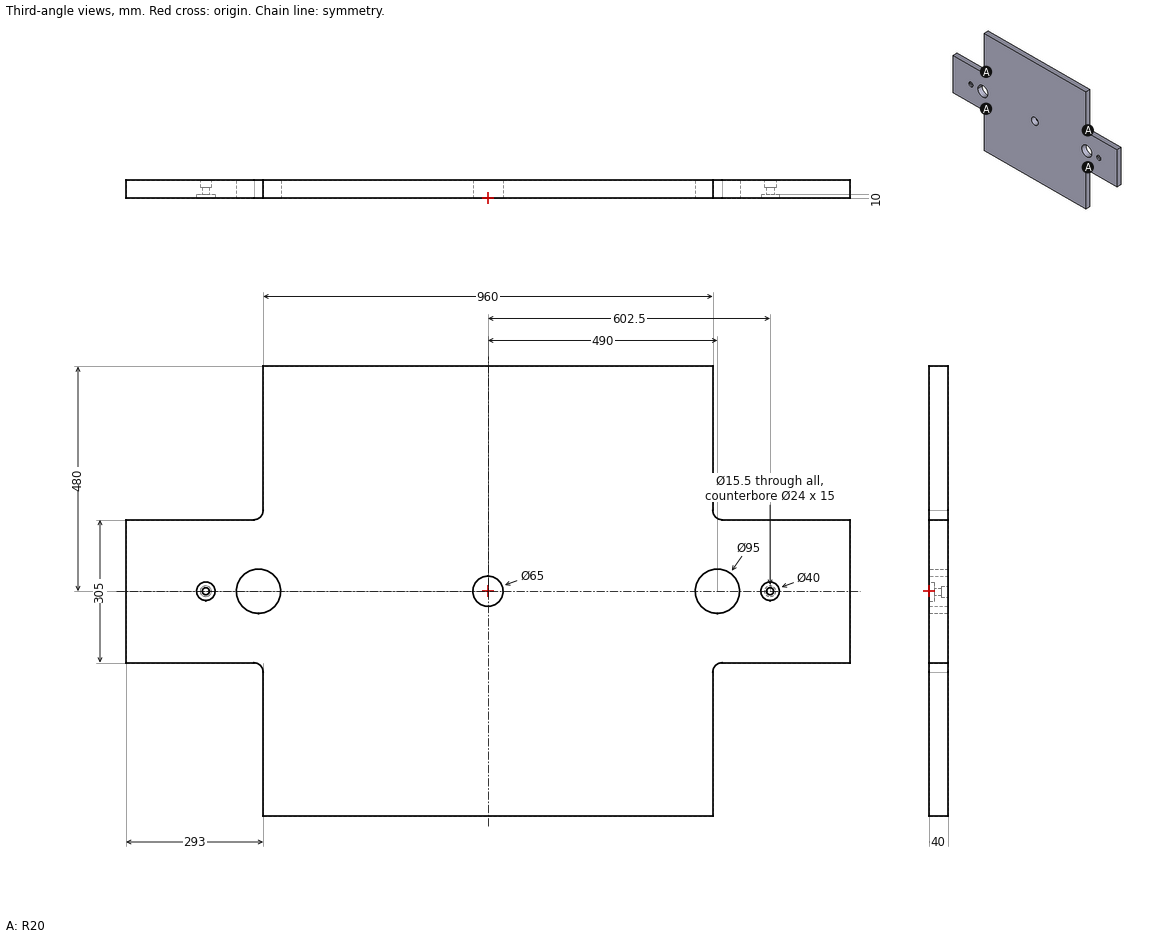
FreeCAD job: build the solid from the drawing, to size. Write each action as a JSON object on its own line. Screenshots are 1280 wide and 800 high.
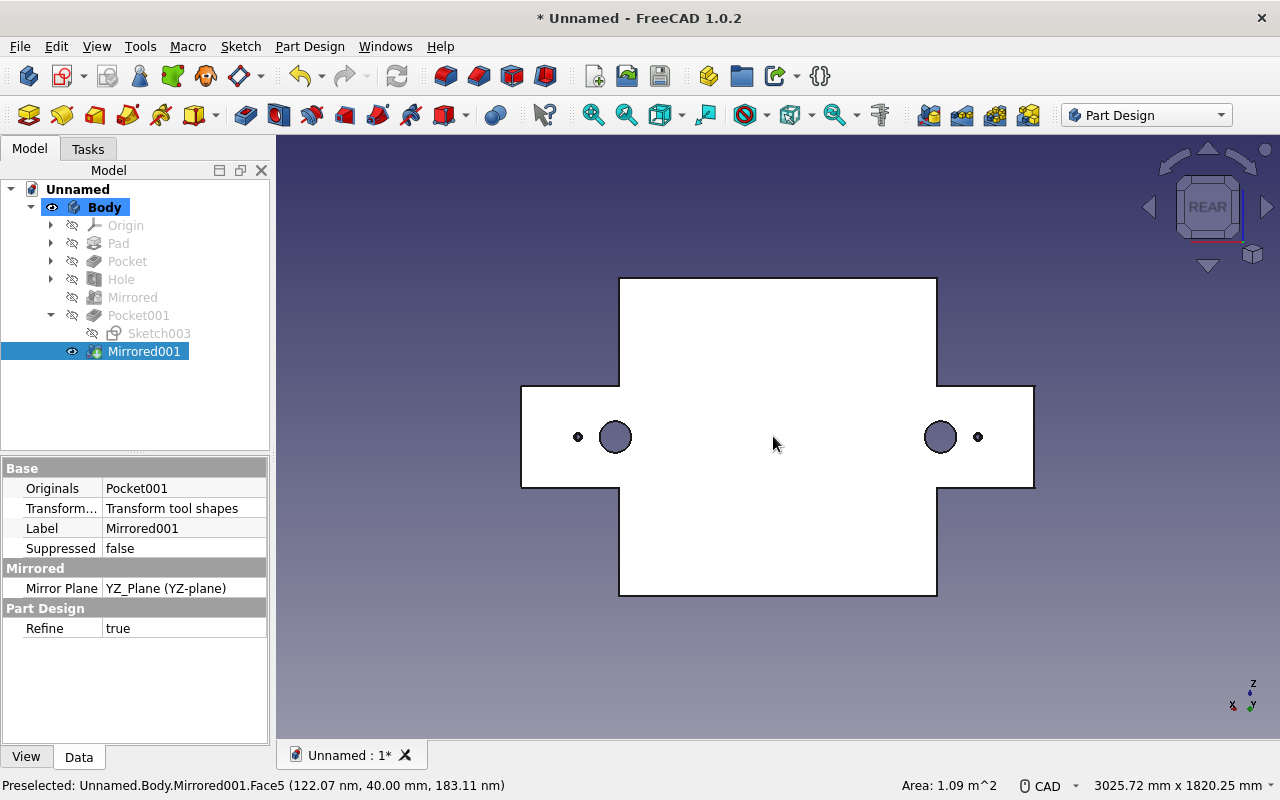
{"action": "left_click", "coordinate": [62, 76]}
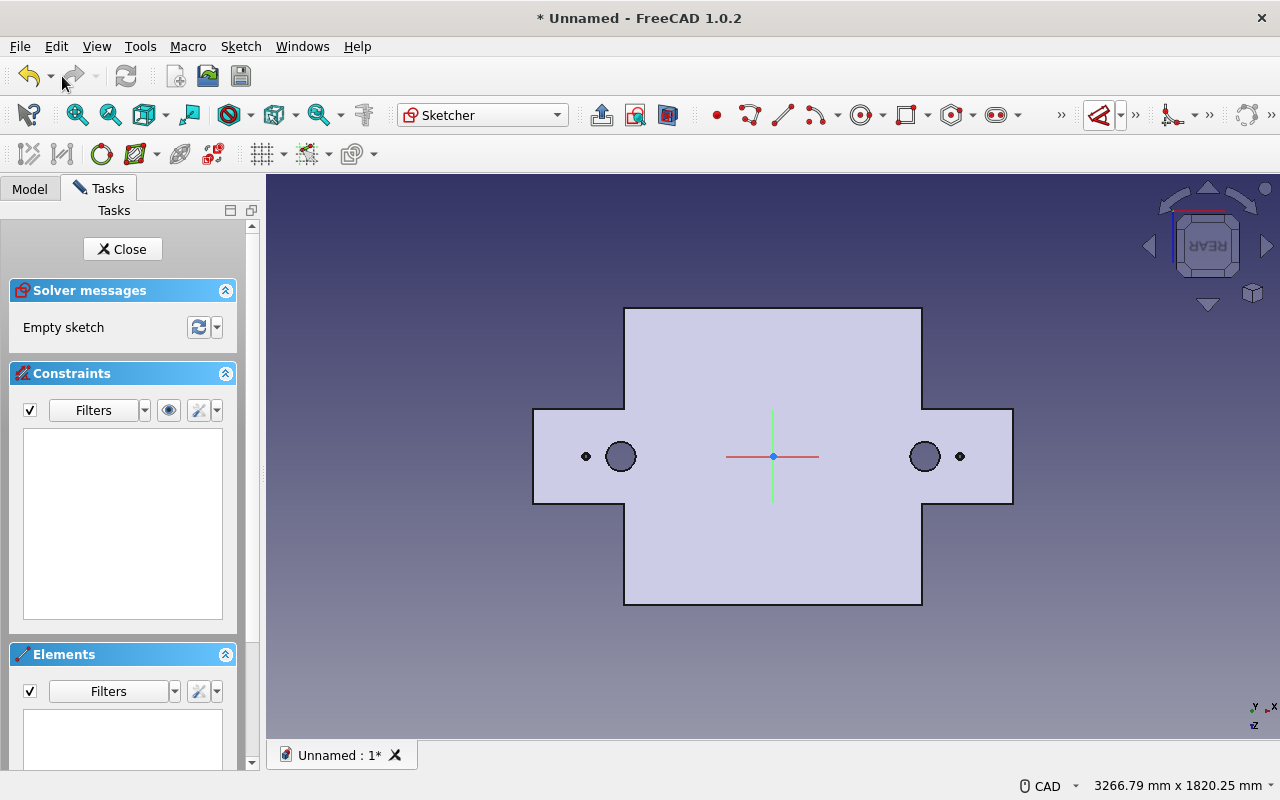
{"action": "scroll", "coordinate": [777, 456], "scroll_direction": "up", "scroll_amount": 14}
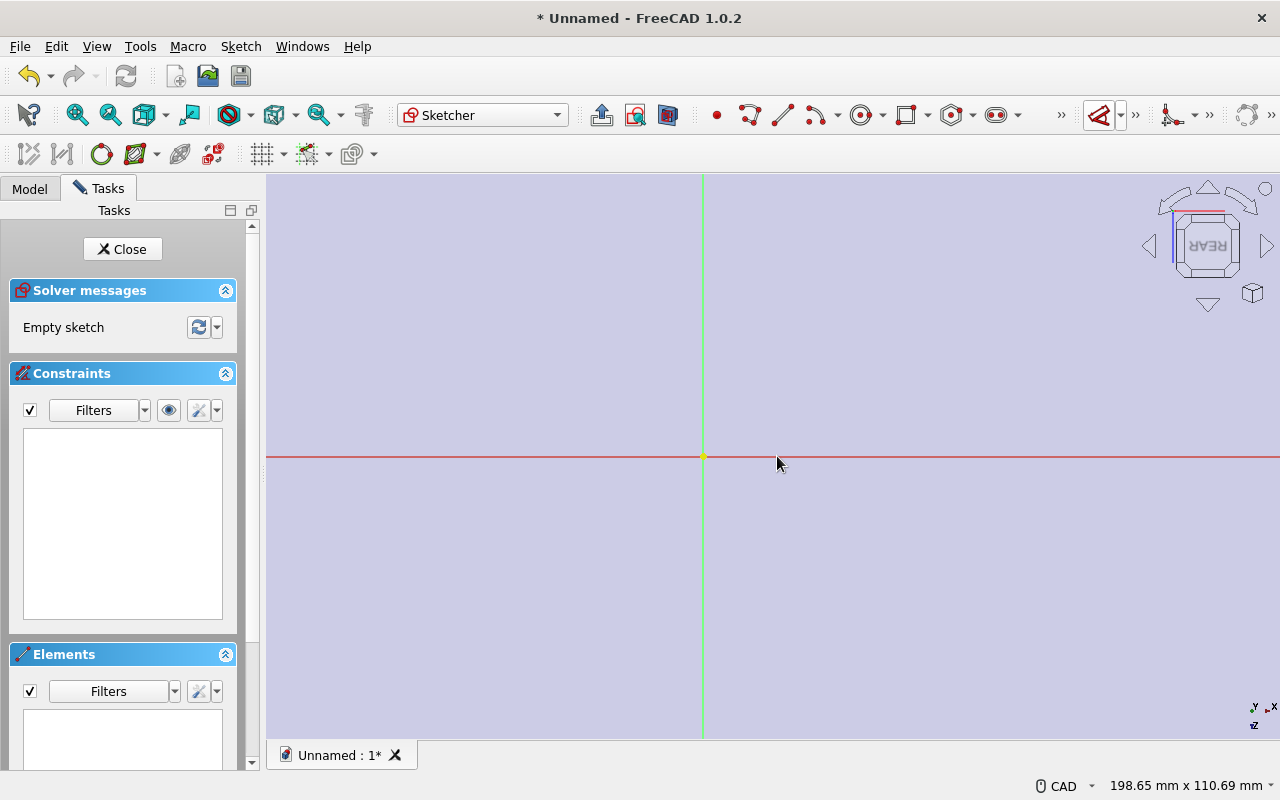
{"action": "left_click", "coordinate": [860, 116]}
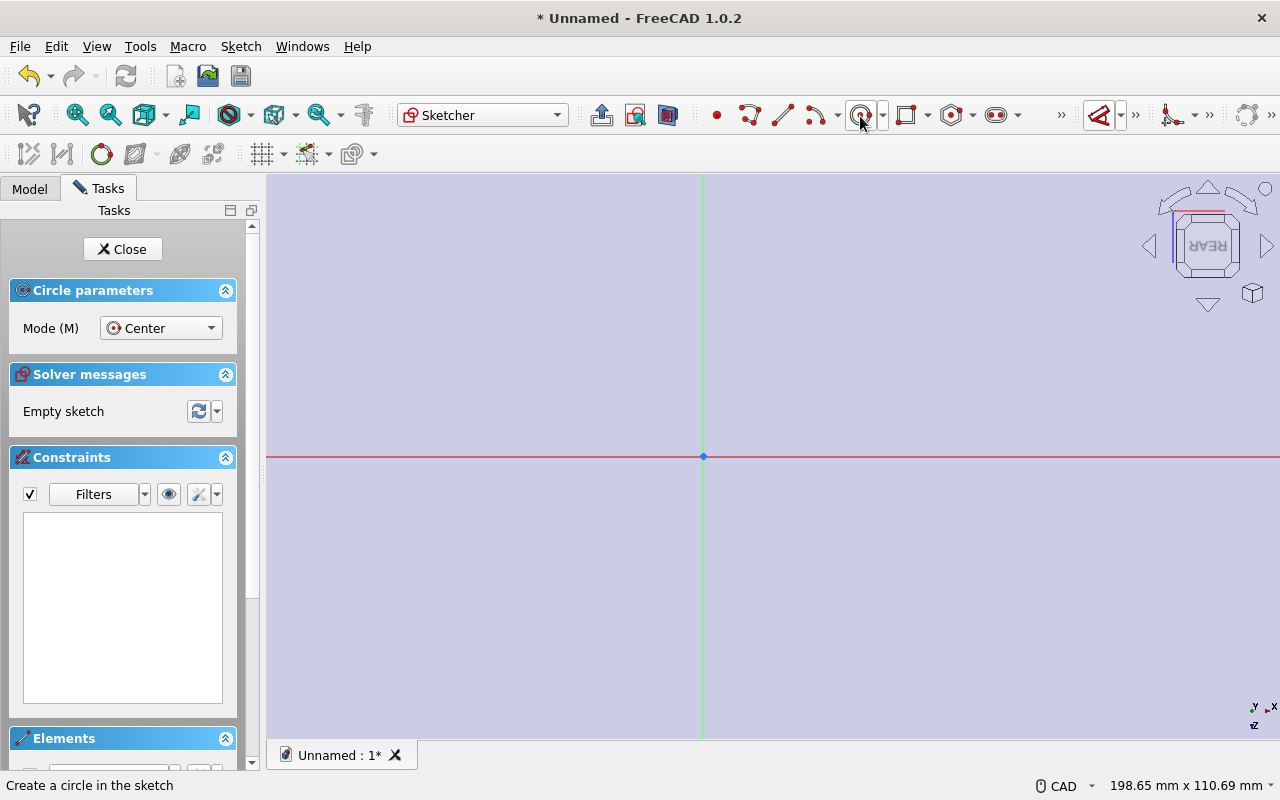
{"action": "left_click", "coordinate": [703, 456]}
{"action": "mouse_move", "coordinate": [821, 339]}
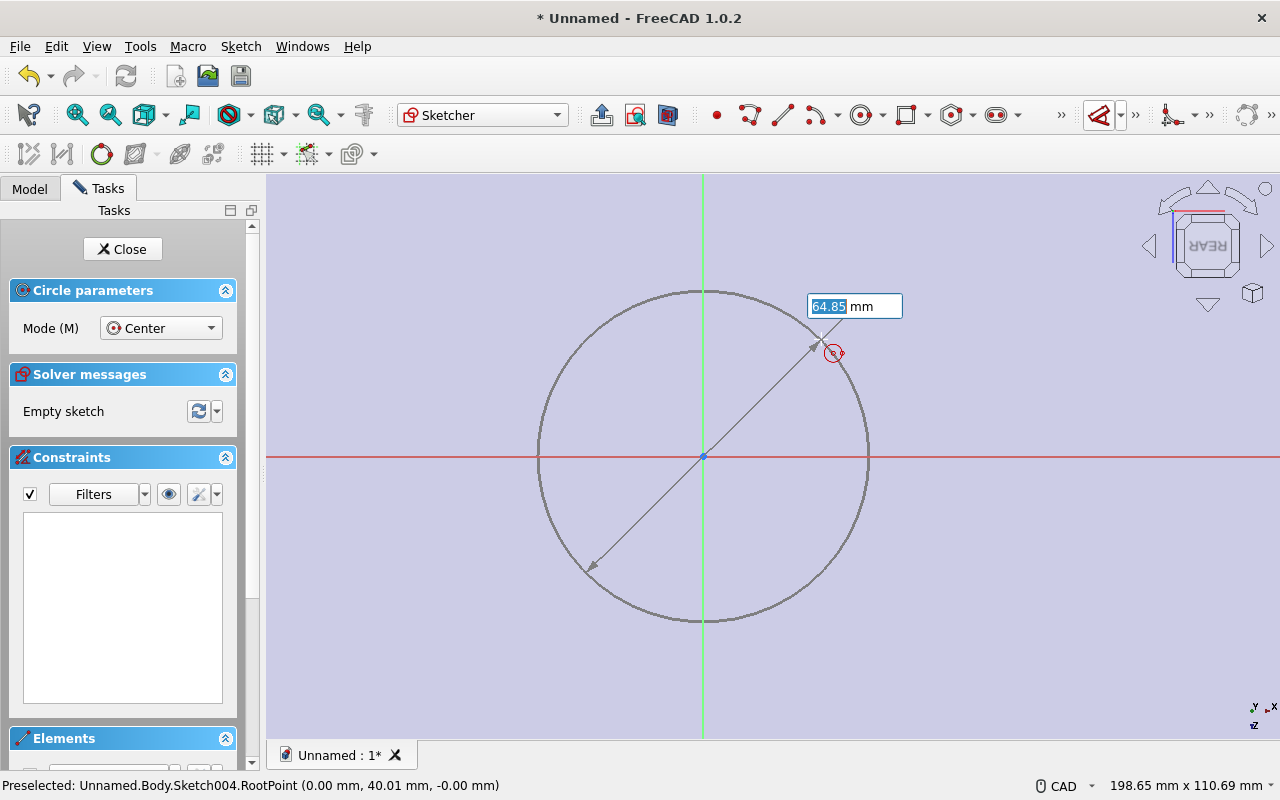
{"action": "type", "text": "65"}
{"action": "key", "text": "Return"}
{"action": "key", "text": "Escape"}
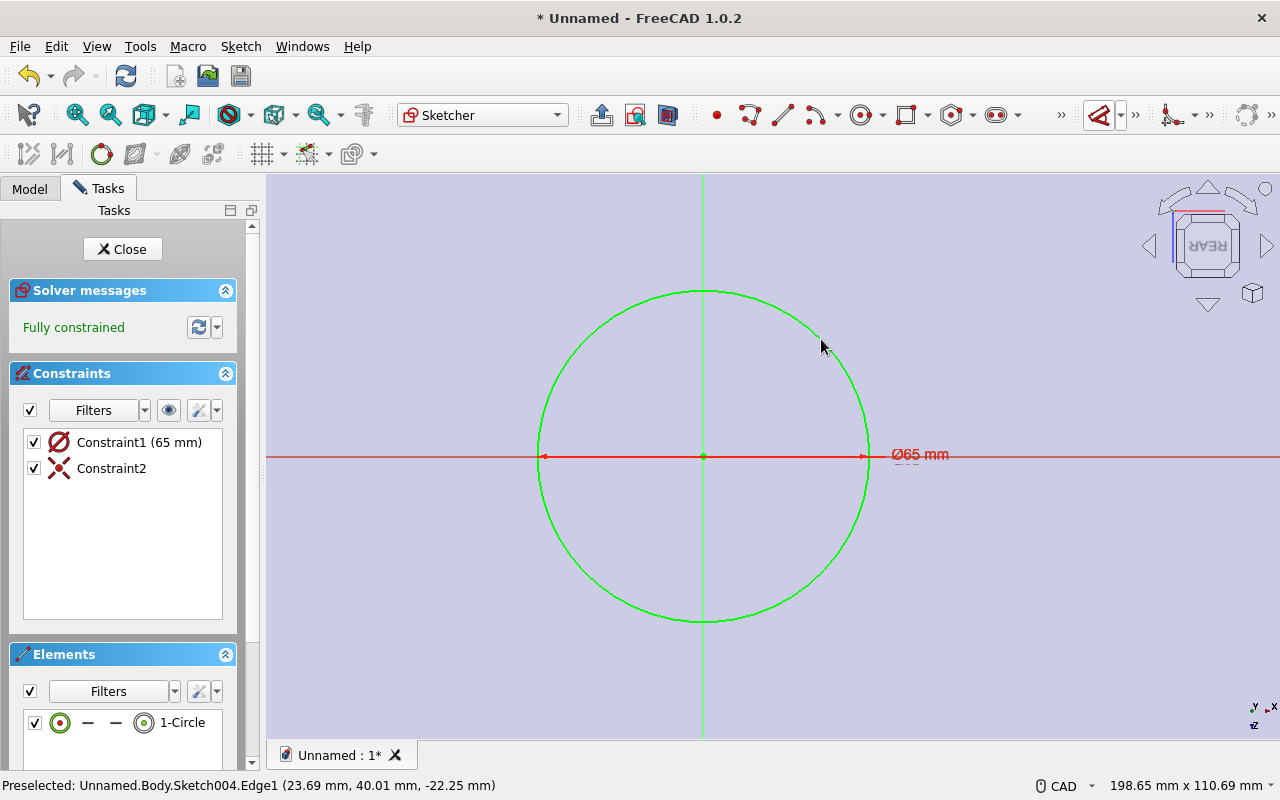
{"action": "left_click", "coordinate": [123, 249]}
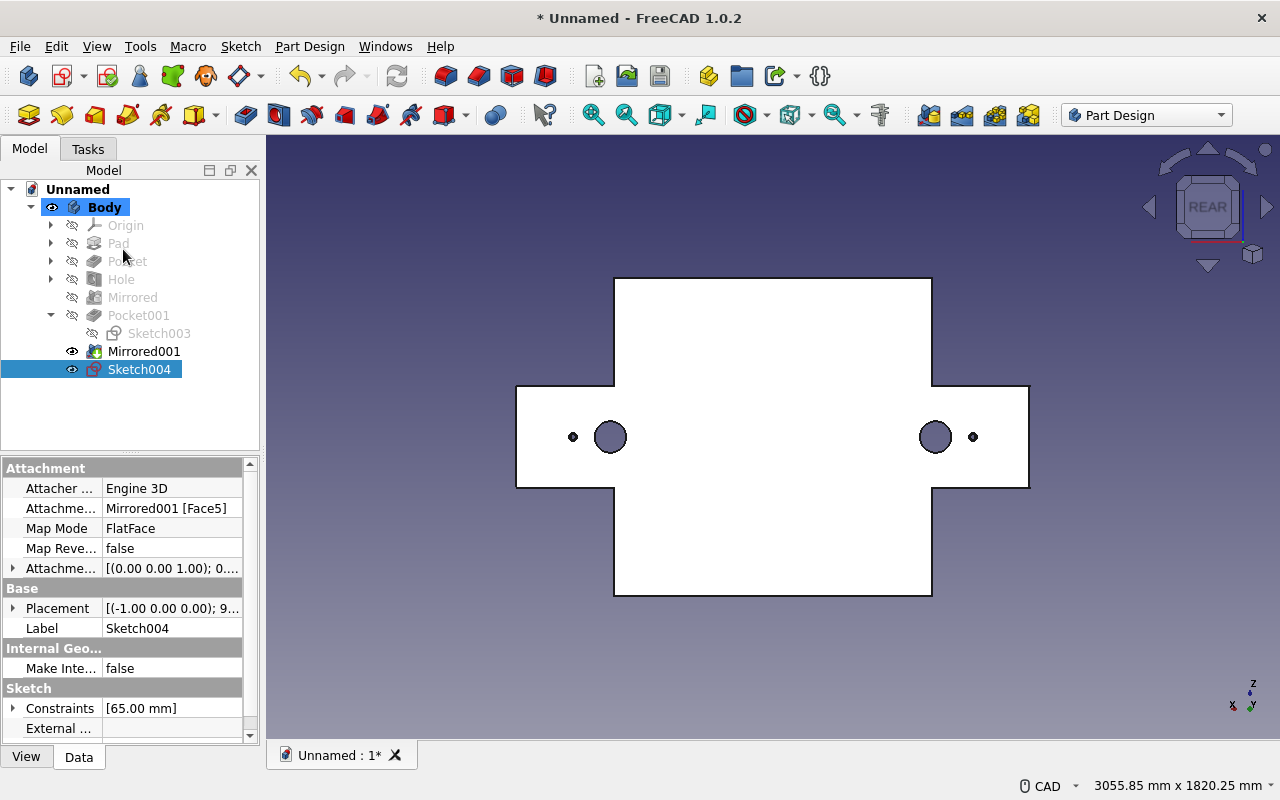
{"action": "left_click", "coordinate": [246, 116]}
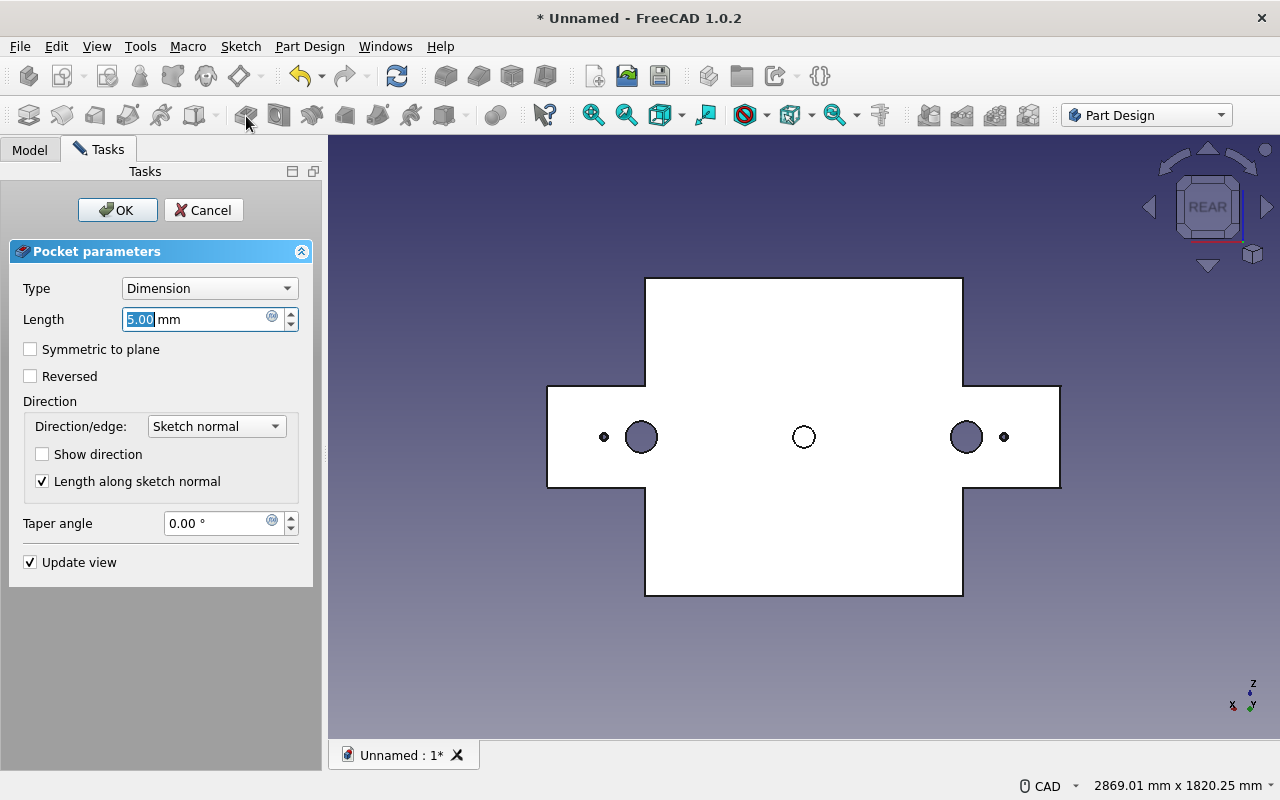
{"action": "left_click", "coordinate": [210, 288]}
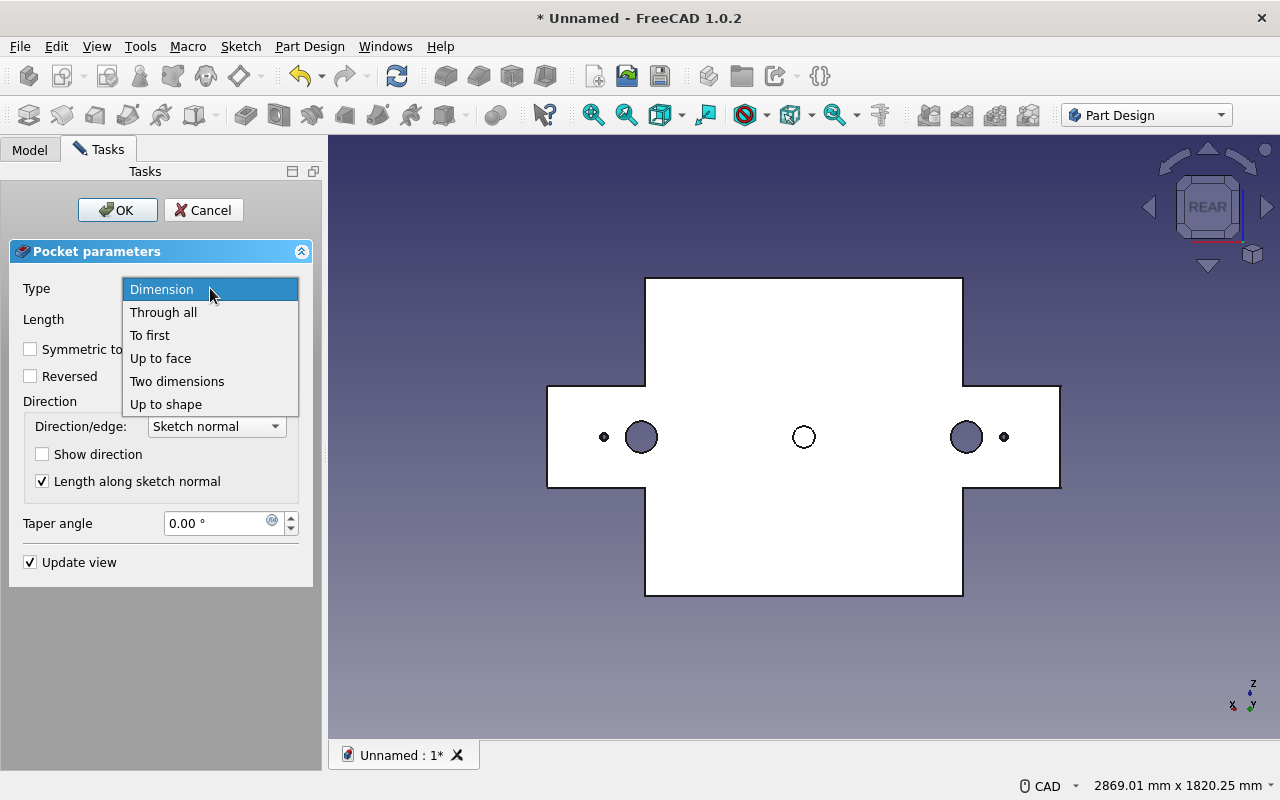
{"action": "left_click", "coordinate": [208, 312]}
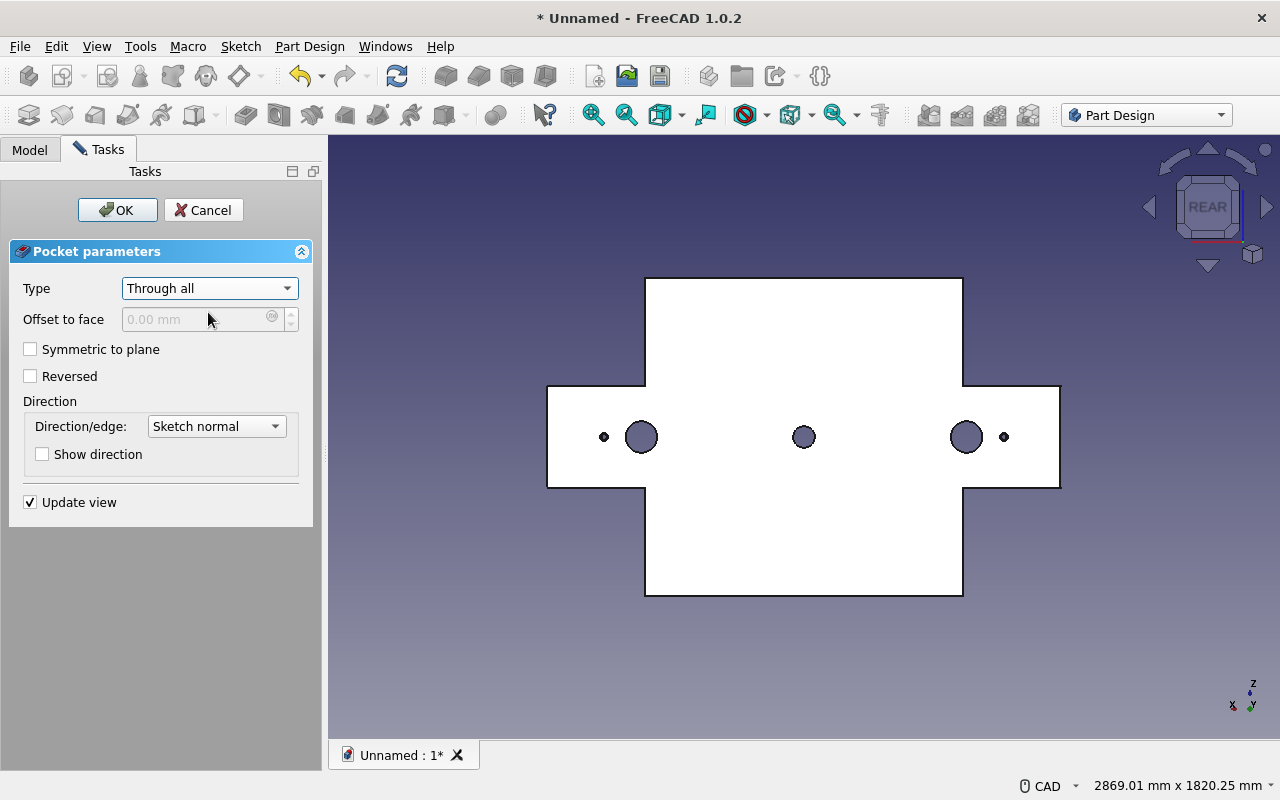
{"action": "left_click", "coordinate": [118, 210]}